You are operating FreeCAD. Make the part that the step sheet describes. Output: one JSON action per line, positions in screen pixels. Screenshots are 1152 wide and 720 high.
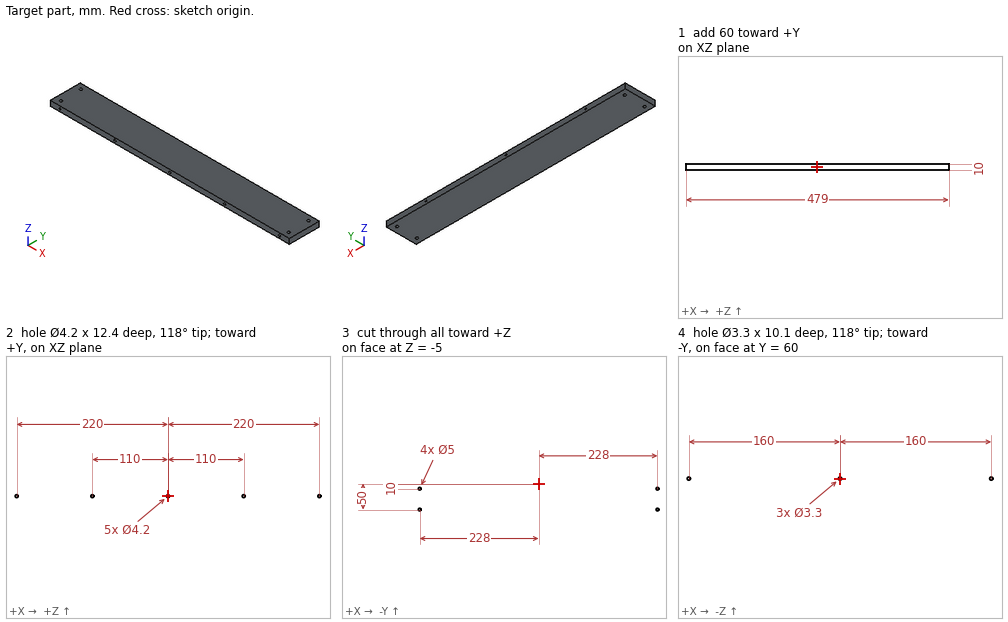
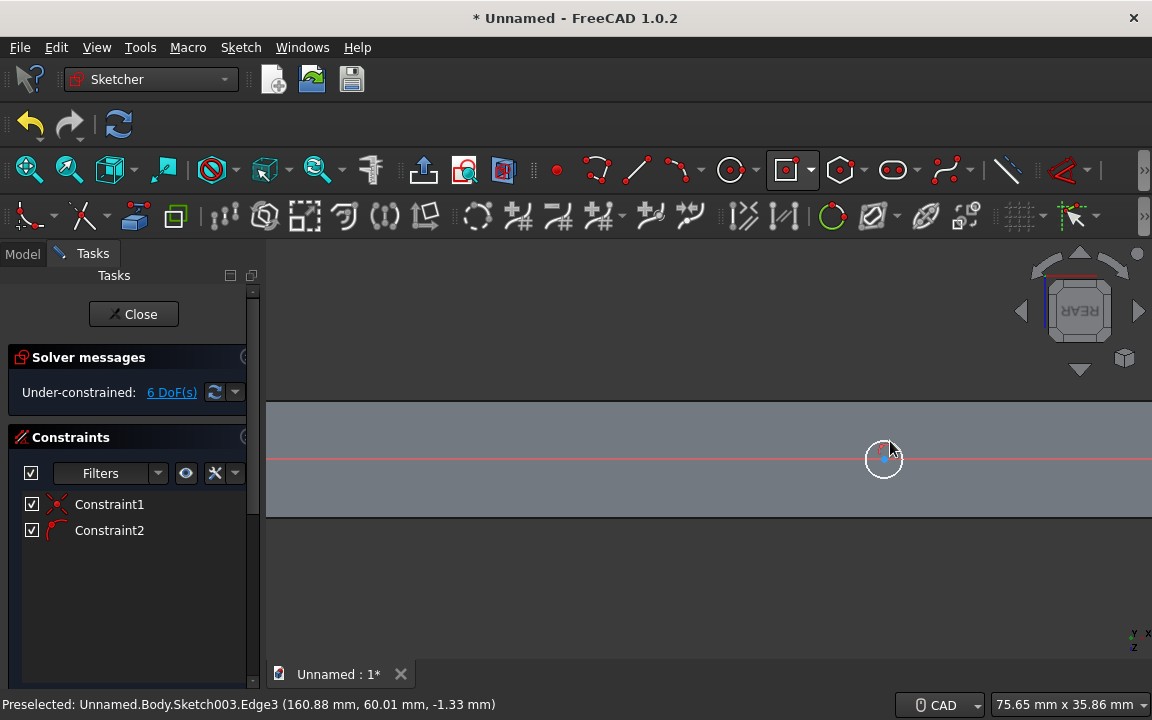
{"action": "scroll", "coordinate": [896, 447], "scroll_direction": "down", "scroll_amount": 10}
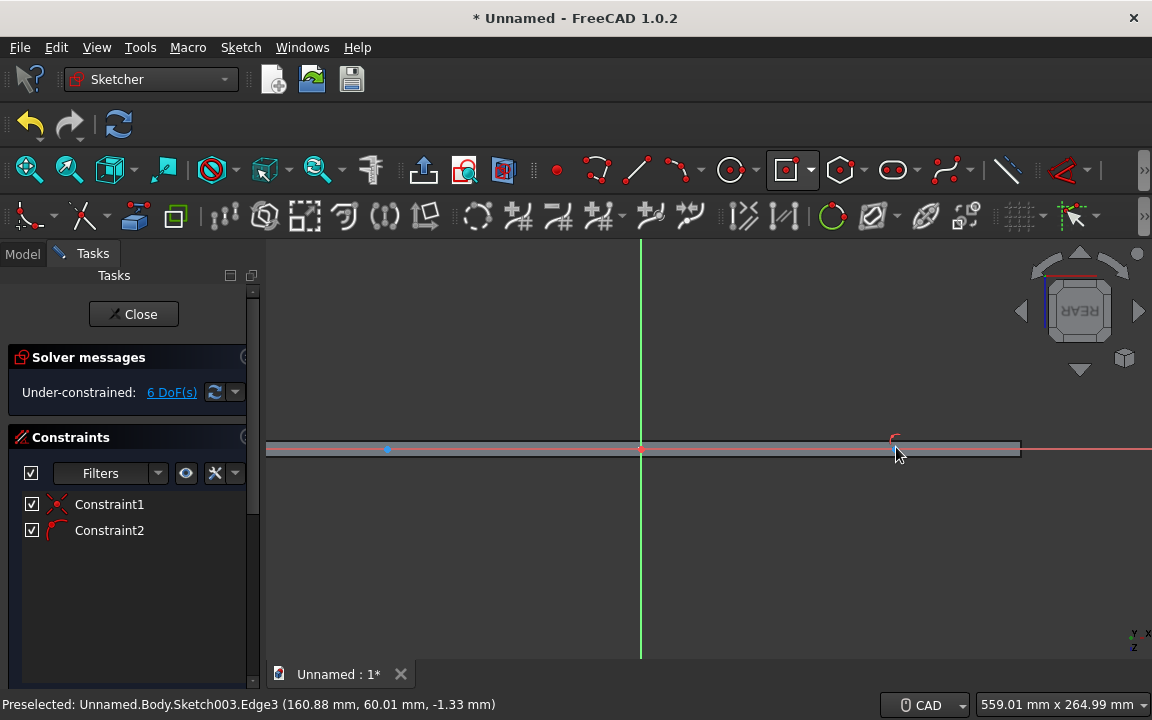
{"action": "scroll", "coordinate": [643, 447], "scroll_direction": "up", "scroll_amount": 11}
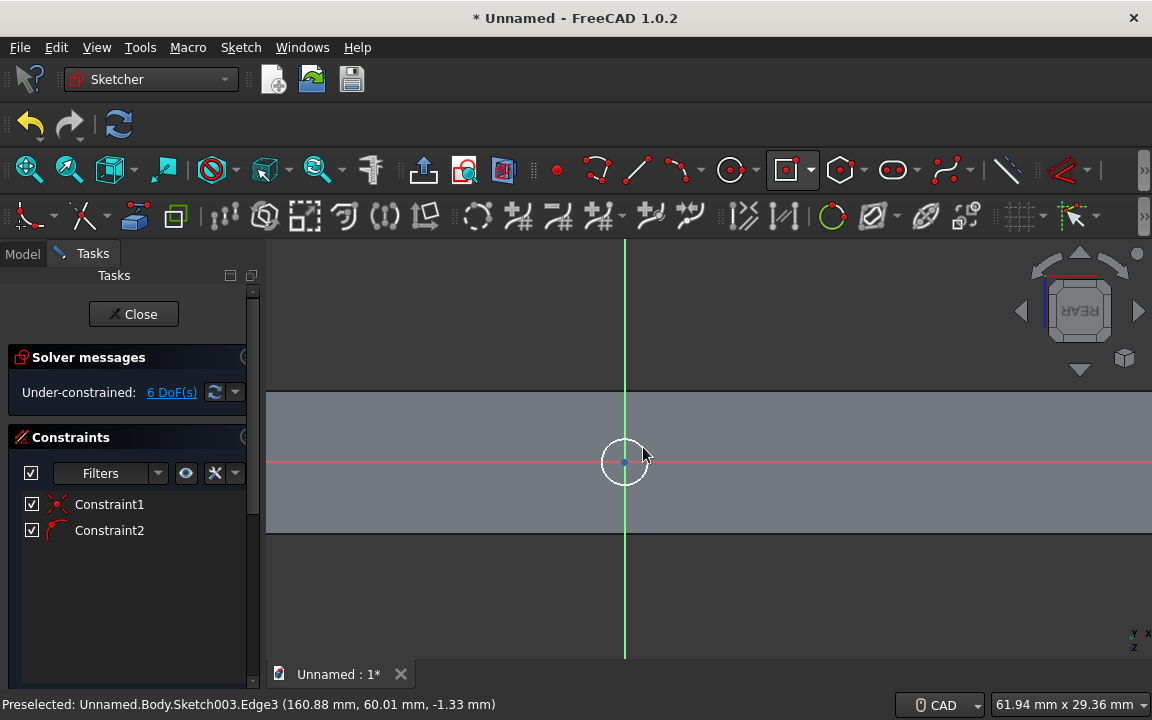
{"action": "left_click", "coordinate": [641, 446]}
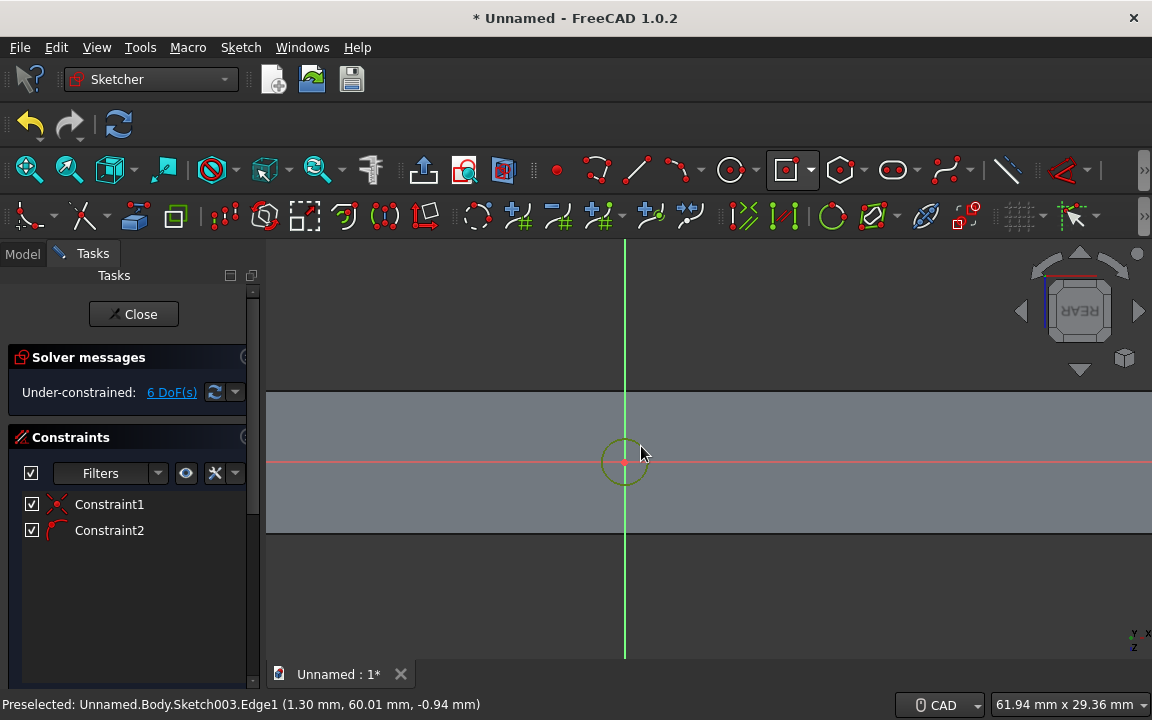
{"action": "scroll", "coordinate": [642, 447], "scroll_direction": "down", "scroll_amount": 11}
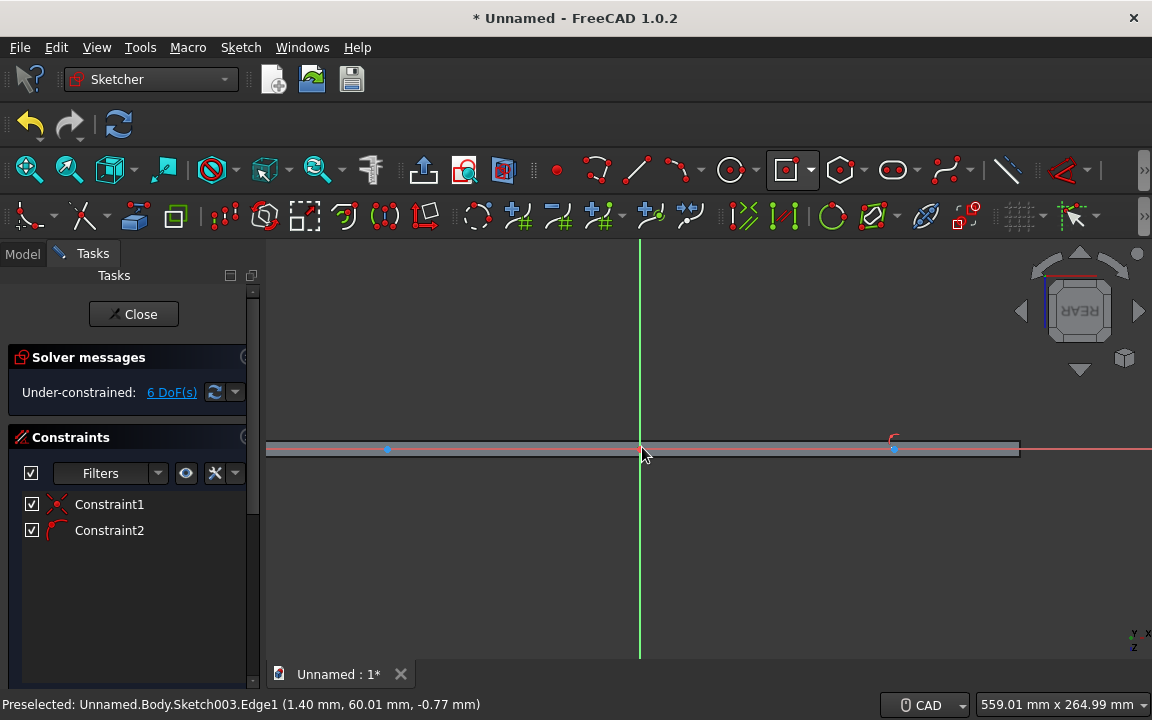
{"action": "scroll", "coordinate": [386, 451], "scroll_direction": "up", "scroll_amount": 10}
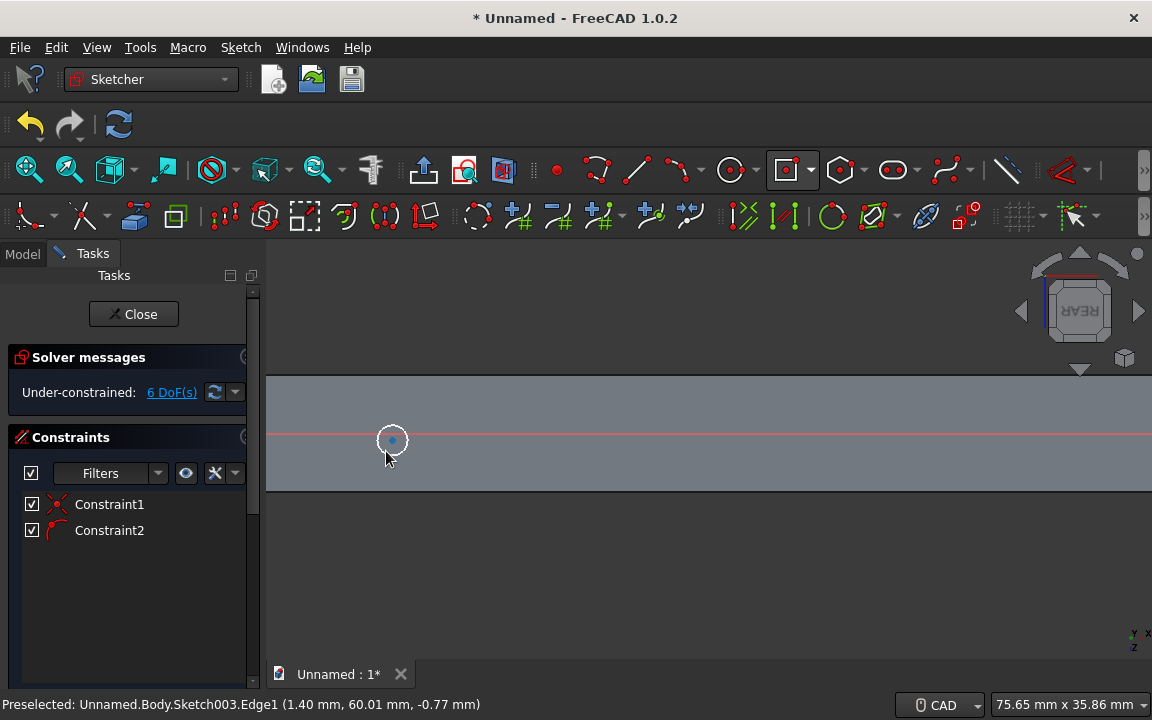
{"action": "left_click", "coordinate": [382, 451]}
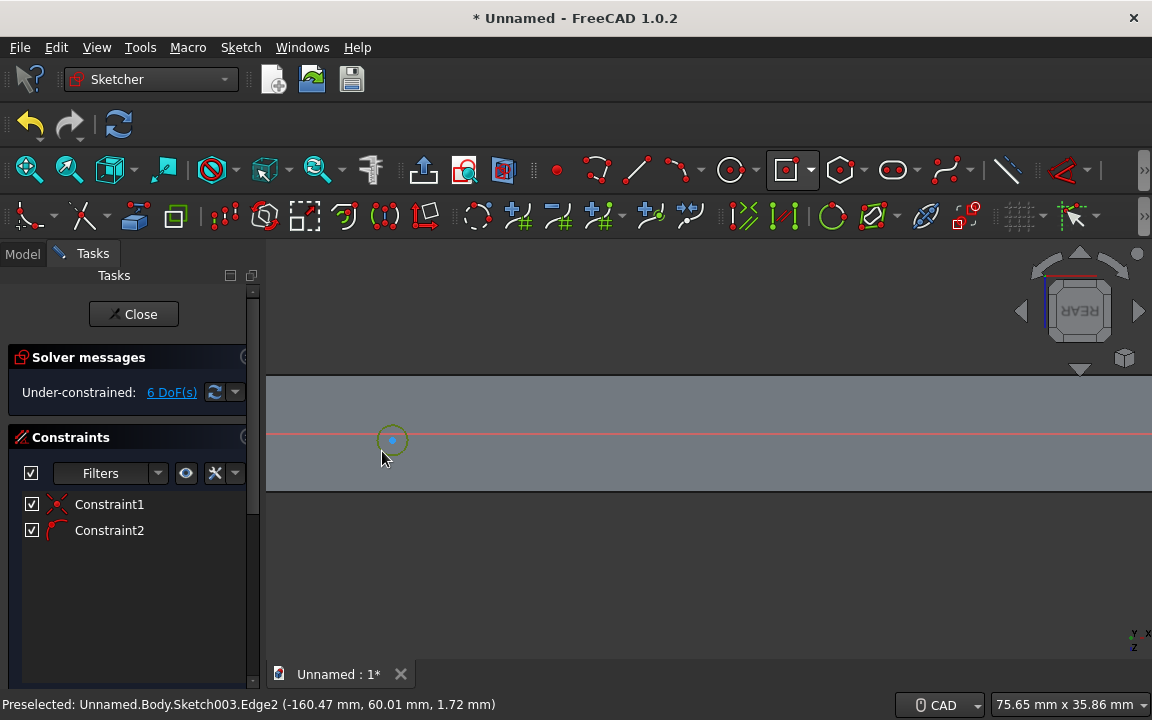
{"action": "scroll", "coordinate": [386, 451], "scroll_direction": "down", "scroll_amount": 10}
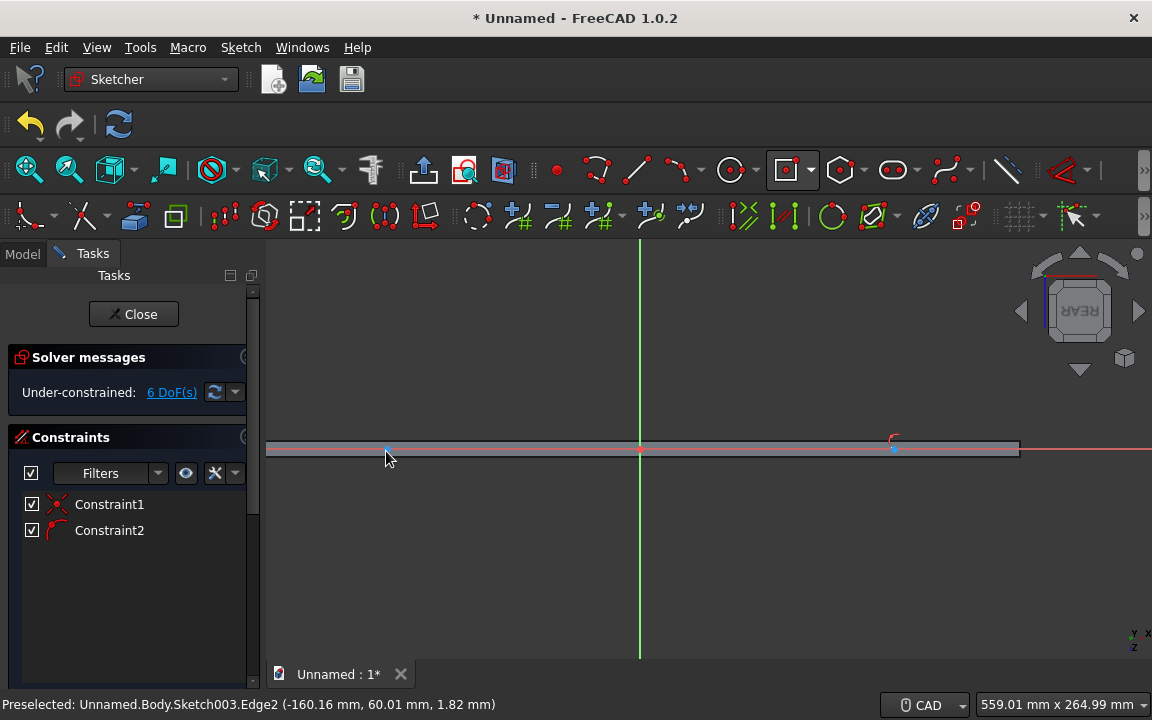
{"action": "scroll", "coordinate": [896, 447], "scroll_direction": "up", "scroll_amount": 11}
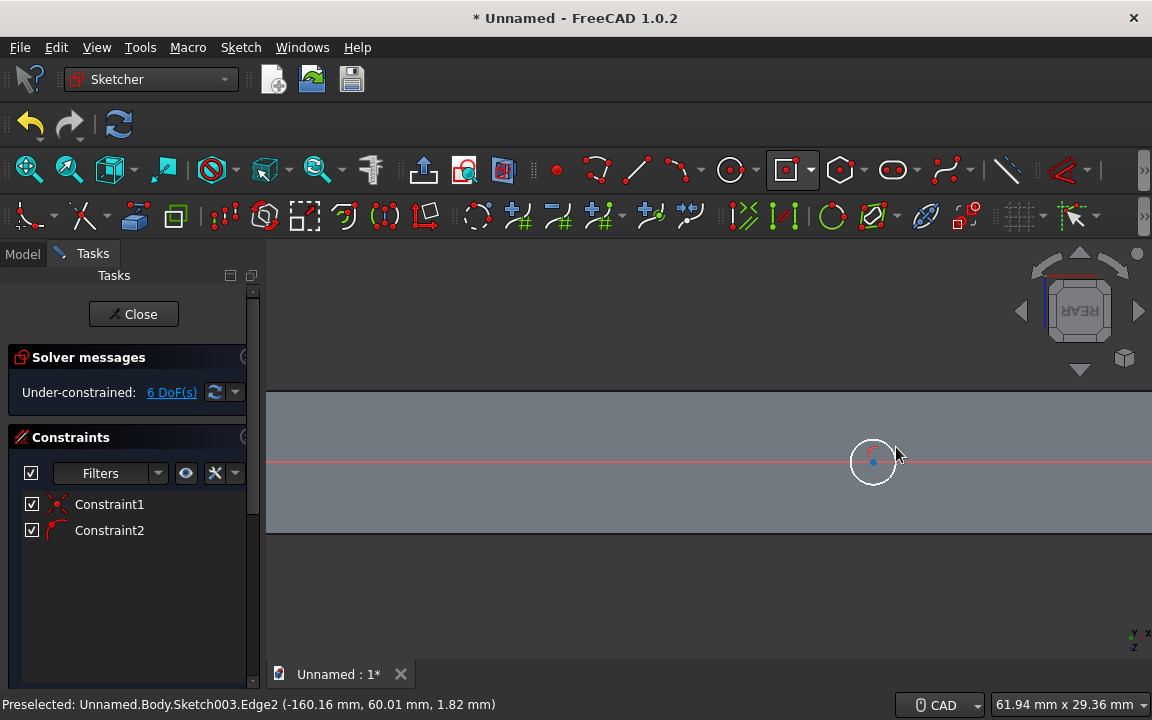
{"action": "left_click", "coordinate": [889, 446]}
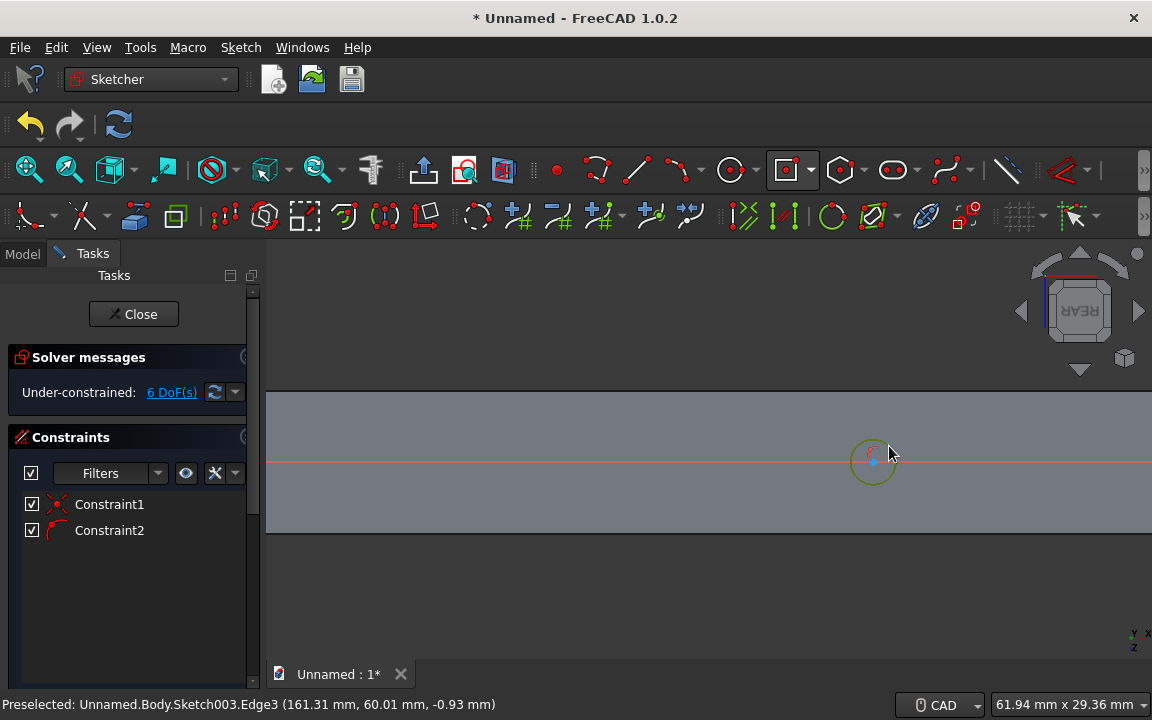
{"action": "key", "text": "e"}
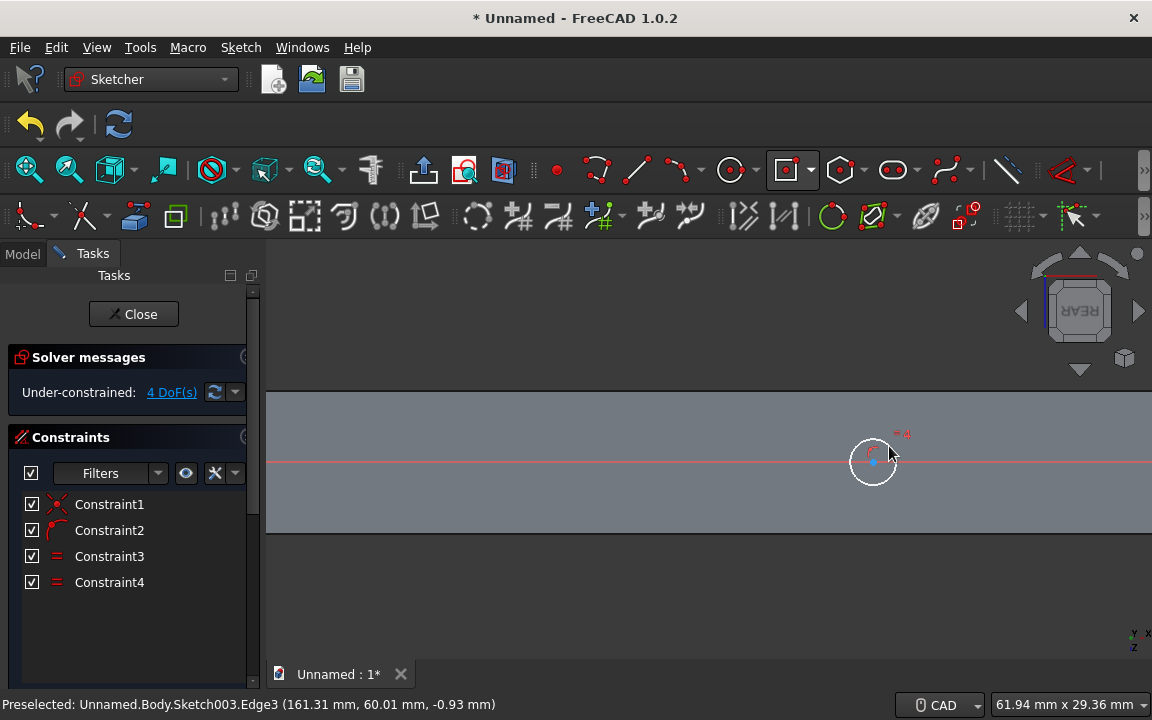
{"action": "scroll", "coordinate": [897, 447], "scroll_direction": "down", "scroll_amount": 11}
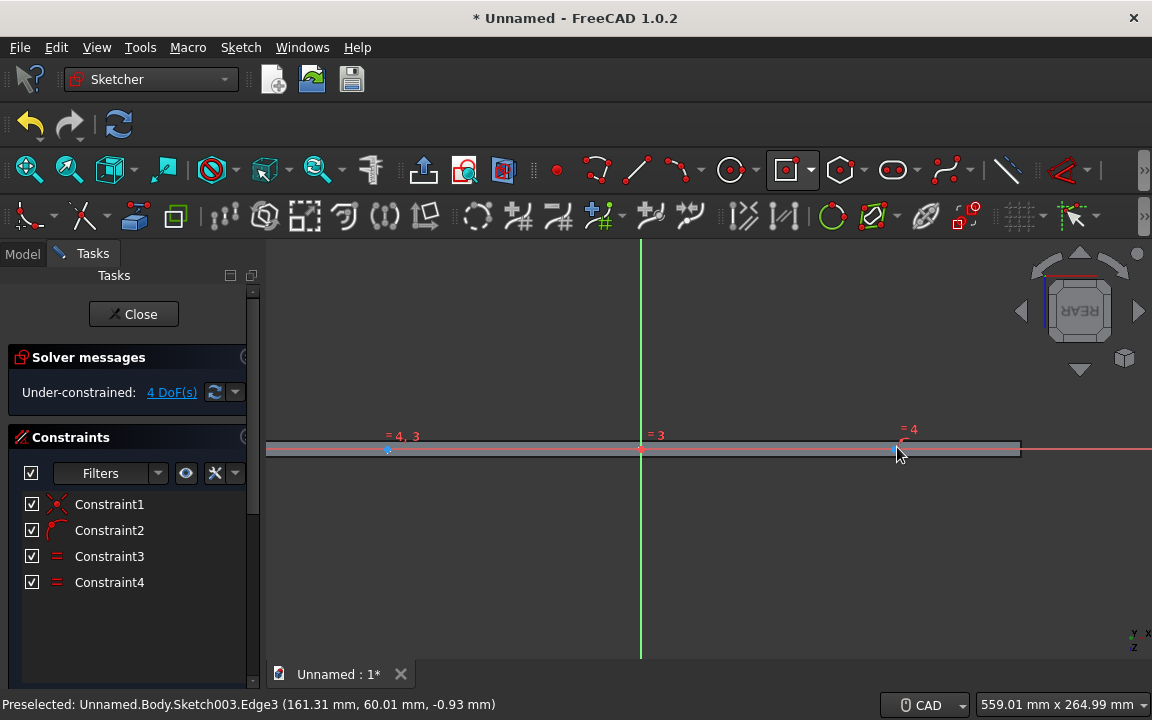
{"action": "left_click", "coordinate": [388, 450]}